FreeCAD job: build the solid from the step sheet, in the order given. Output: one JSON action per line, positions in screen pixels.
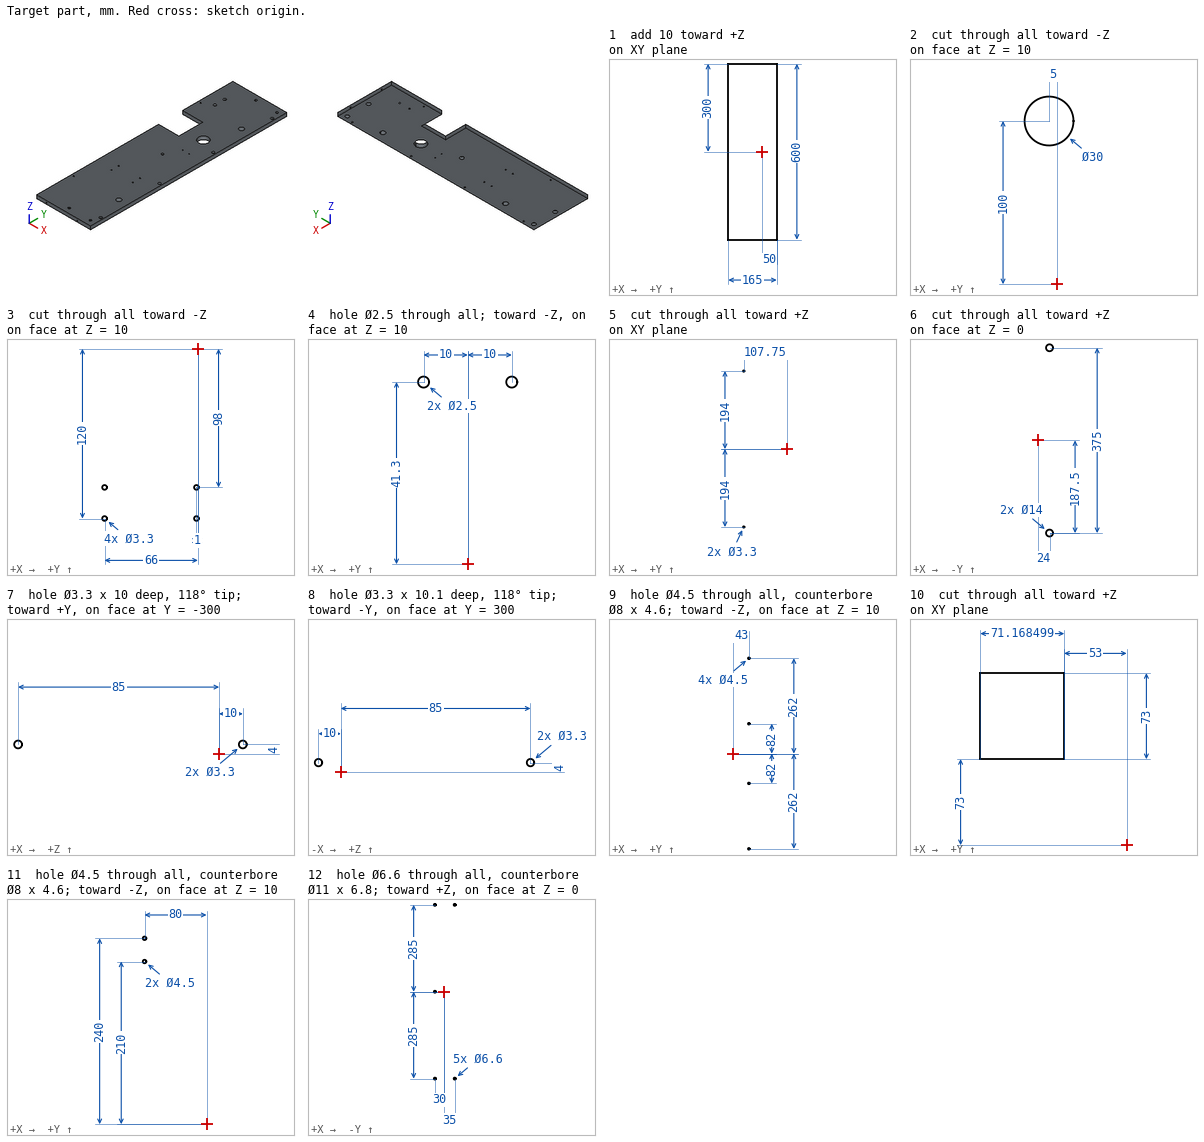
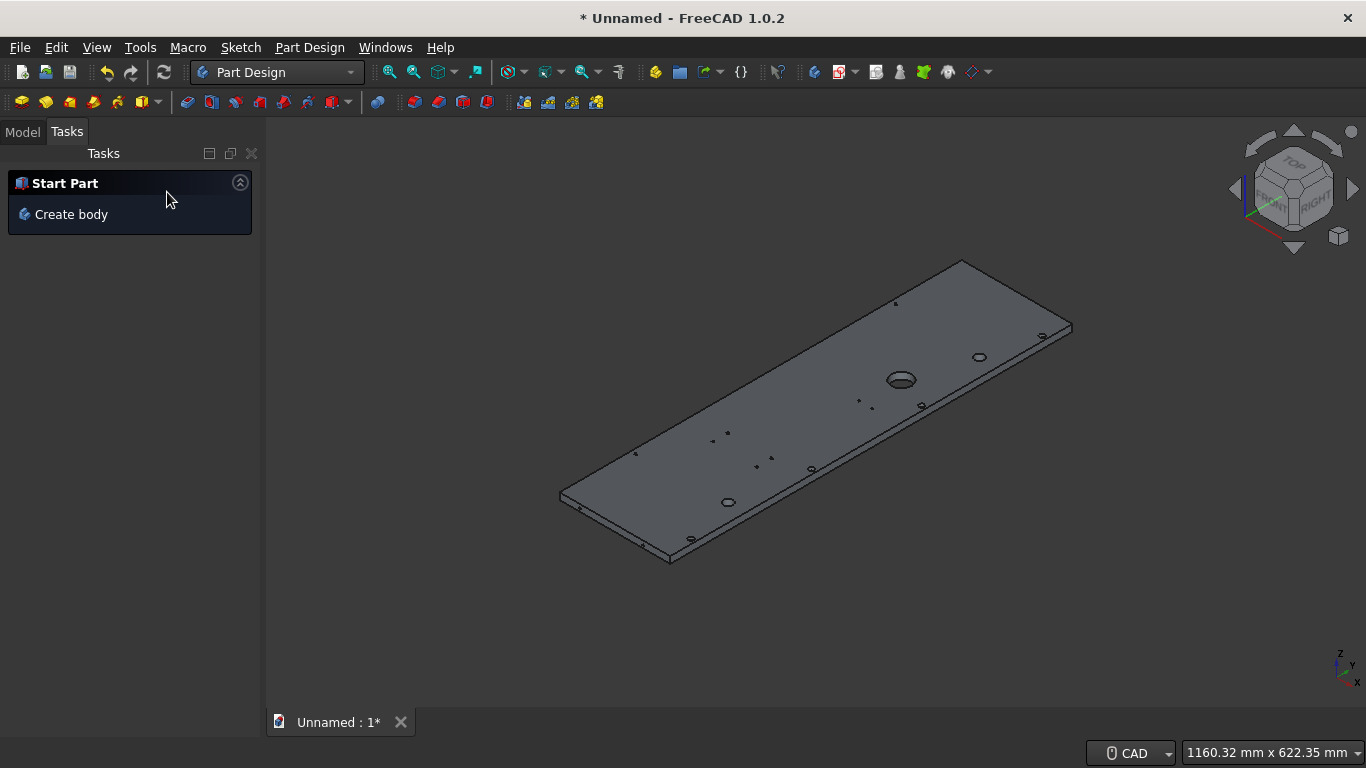
{"action": "left_click", "coordinate": [840, 72]}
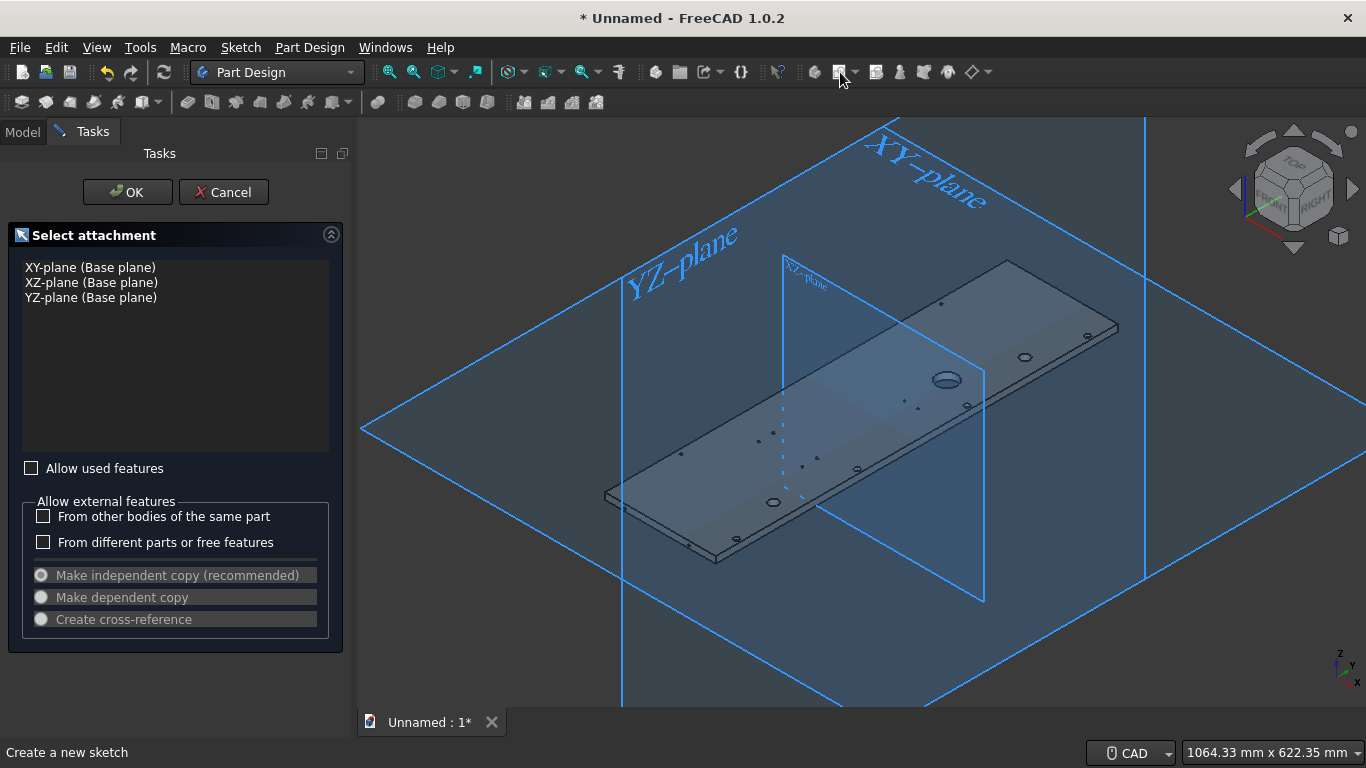
{"action": "left_click", "coordinate": [82, 268]}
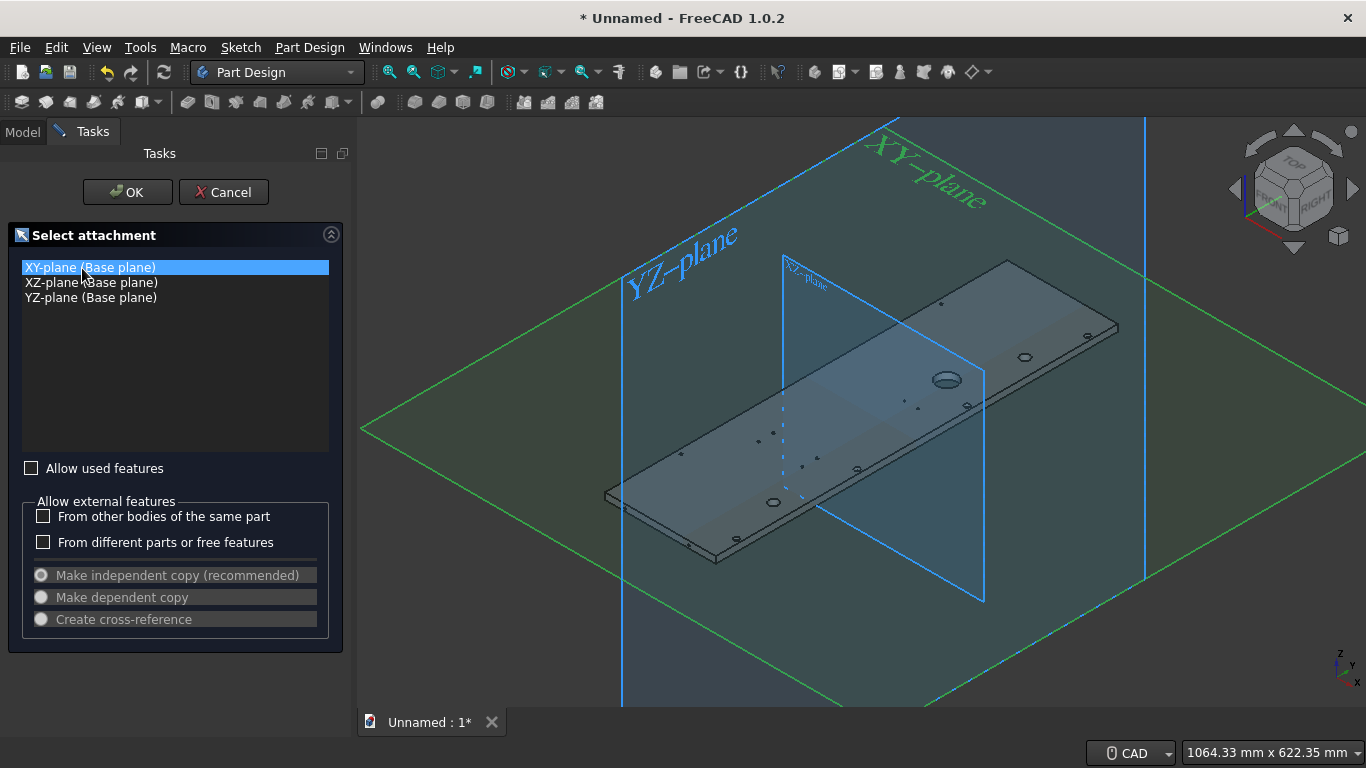
{"action": "left_click", "coordinate": [128, 192]}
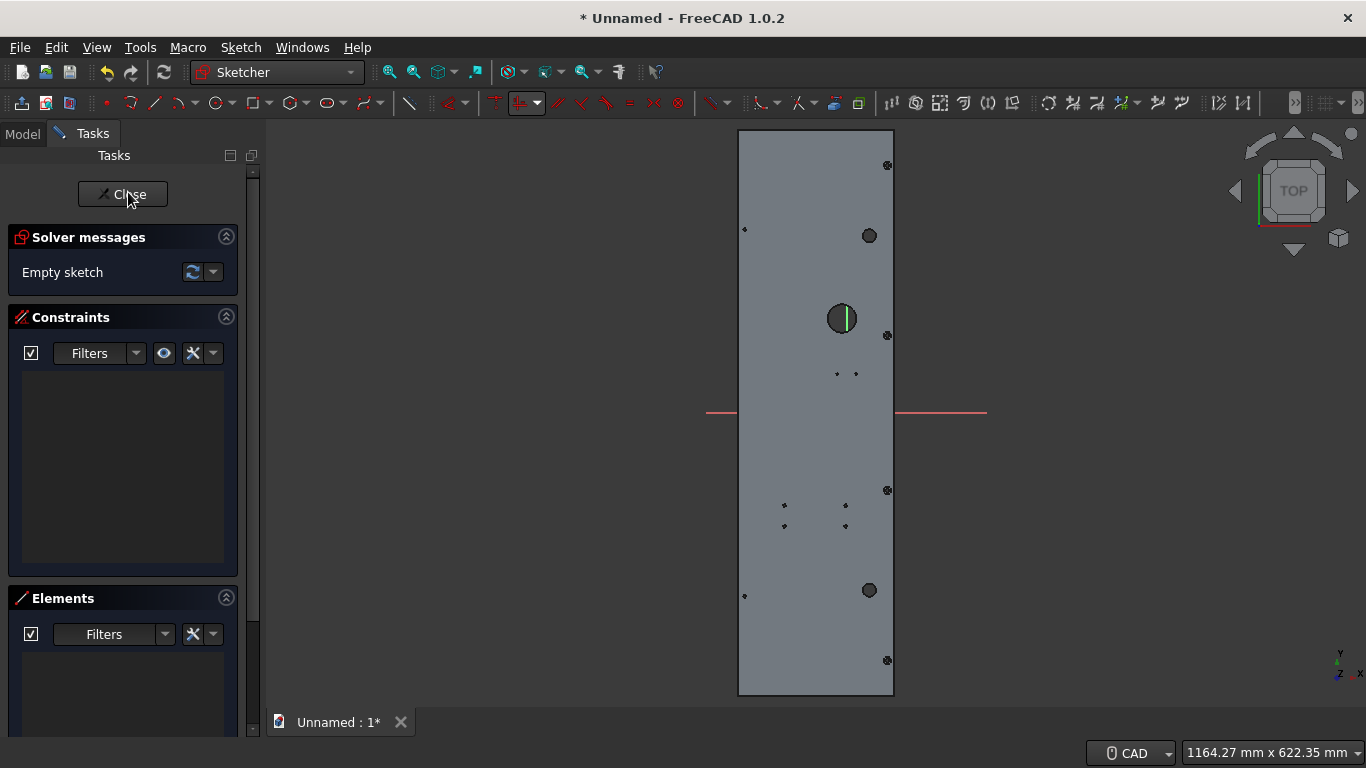
{"action": "left_click", "coordinate": [70, 104]}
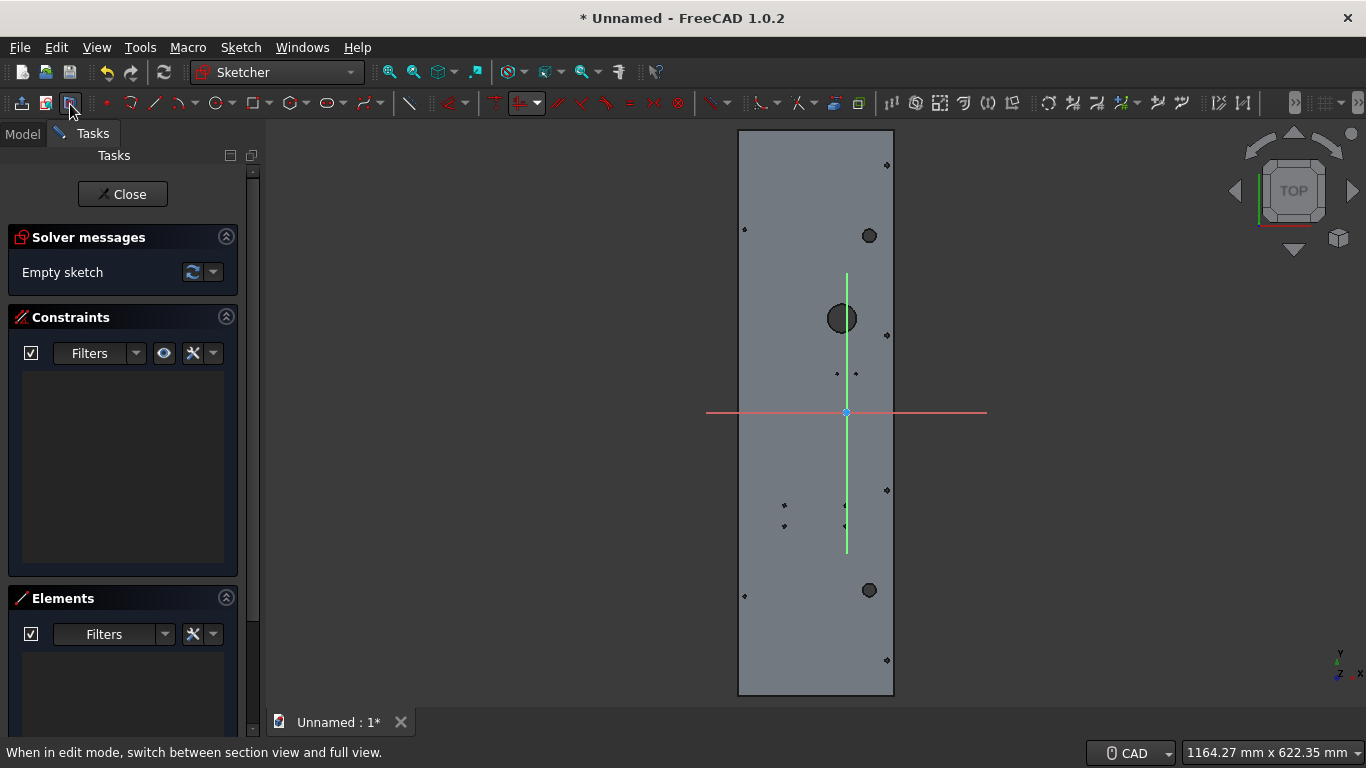
{"action": "scroll", "coordinate": [812, 304], "scroll_direction": "up", "scroll_amount": 5}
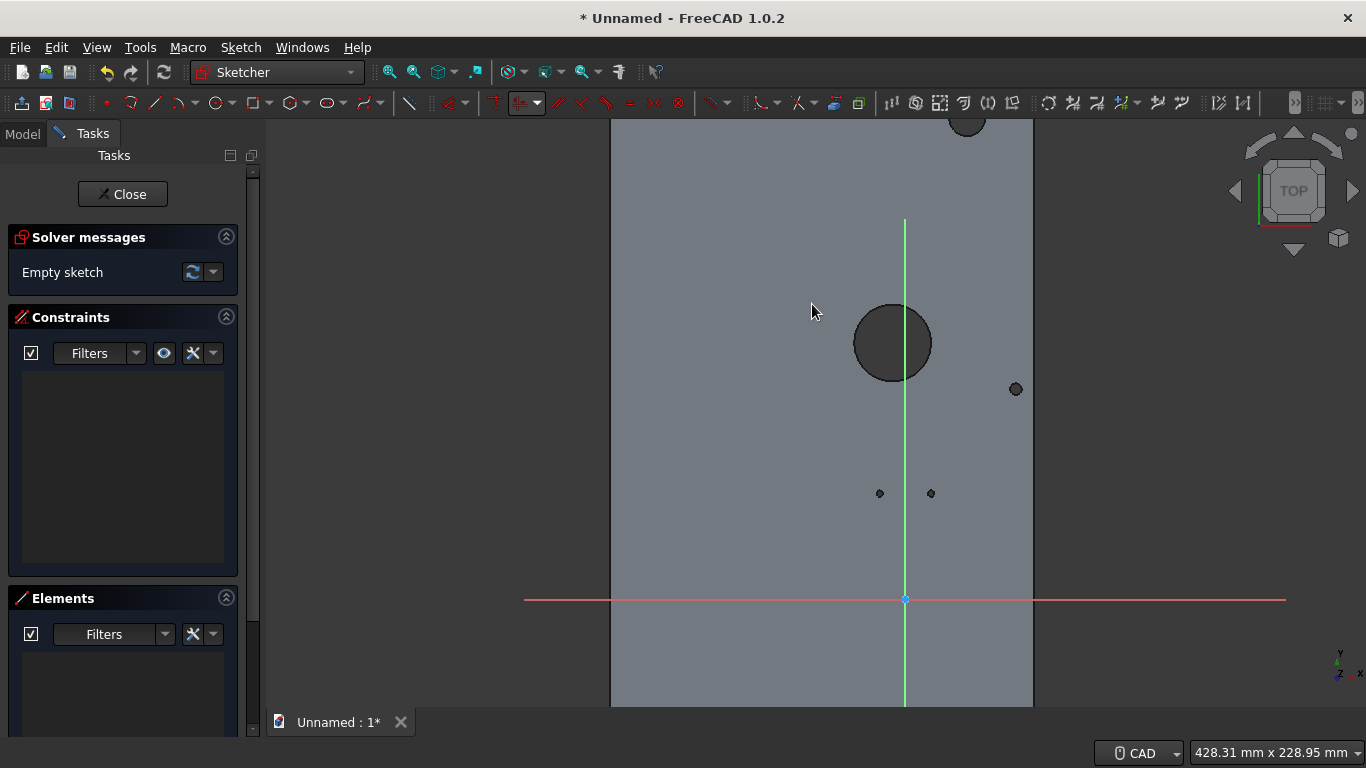
{"action": "left_click", "coordinate": [254, 104]}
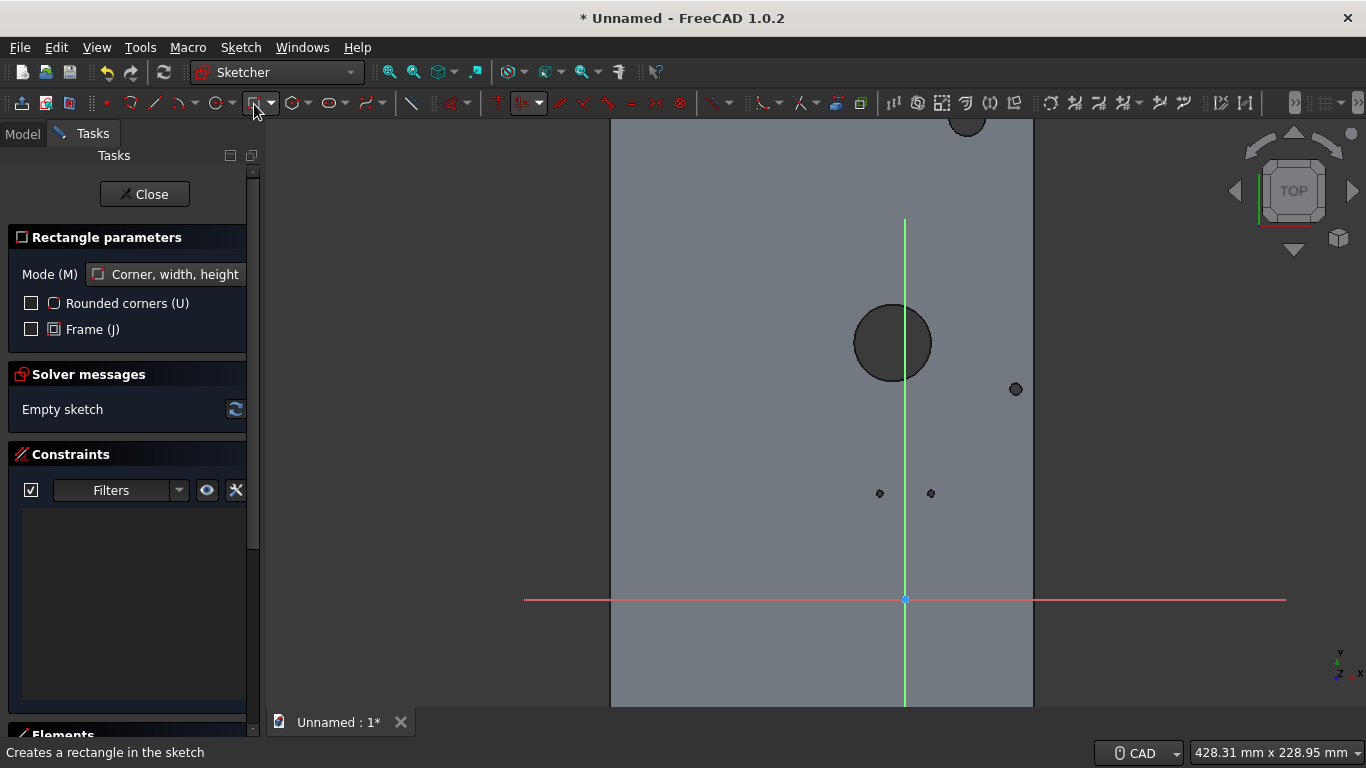
{"action": "left_click", "coordinate": [587, 225]}
{"action": "mouse_move", "coordinate": [769, 412]}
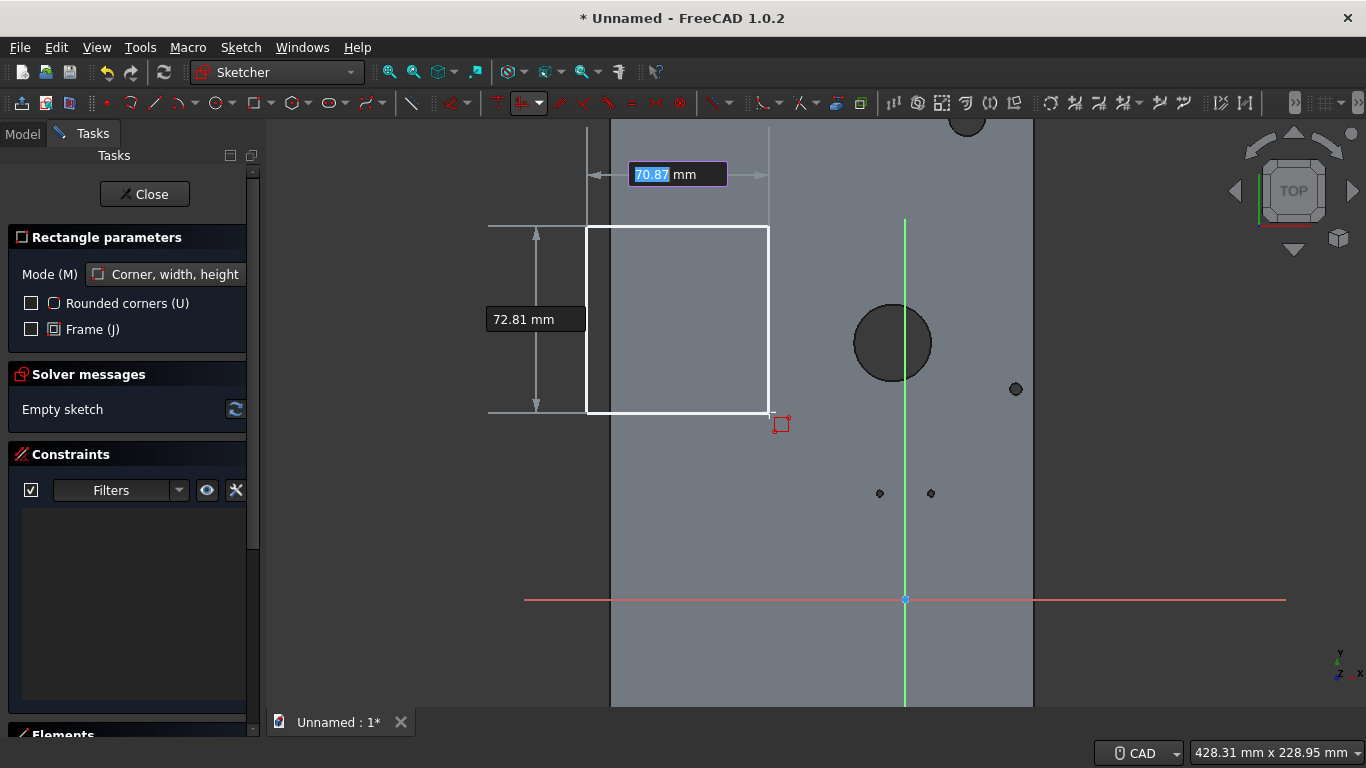
{"action": "type", "text": "71.168499"}
{"action": "key", "text": "Tab"}
{"action": "type", "text": "73"}
{"action": "key", "text": "Return"}
{"action": "key", "text": "Escape"}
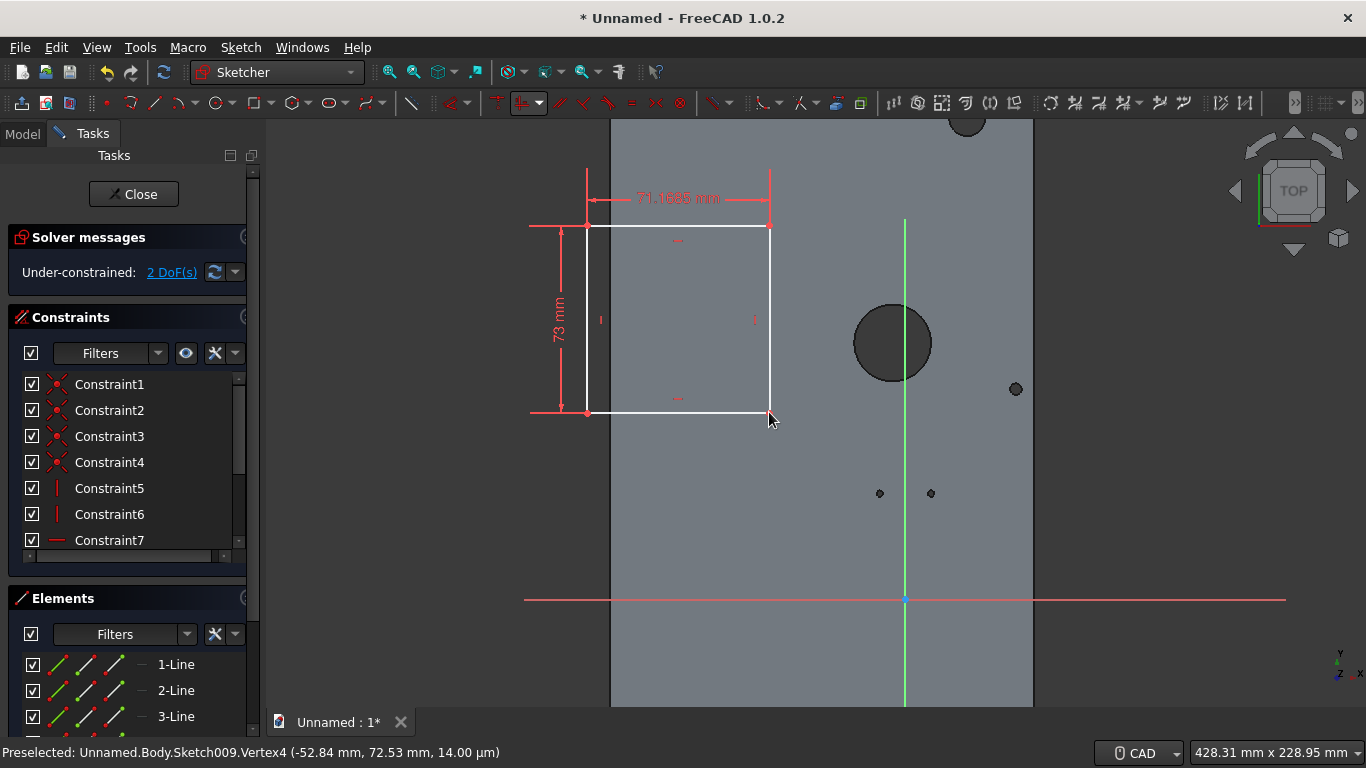
{"action": "left_click", "coordinate": [450, 104]}